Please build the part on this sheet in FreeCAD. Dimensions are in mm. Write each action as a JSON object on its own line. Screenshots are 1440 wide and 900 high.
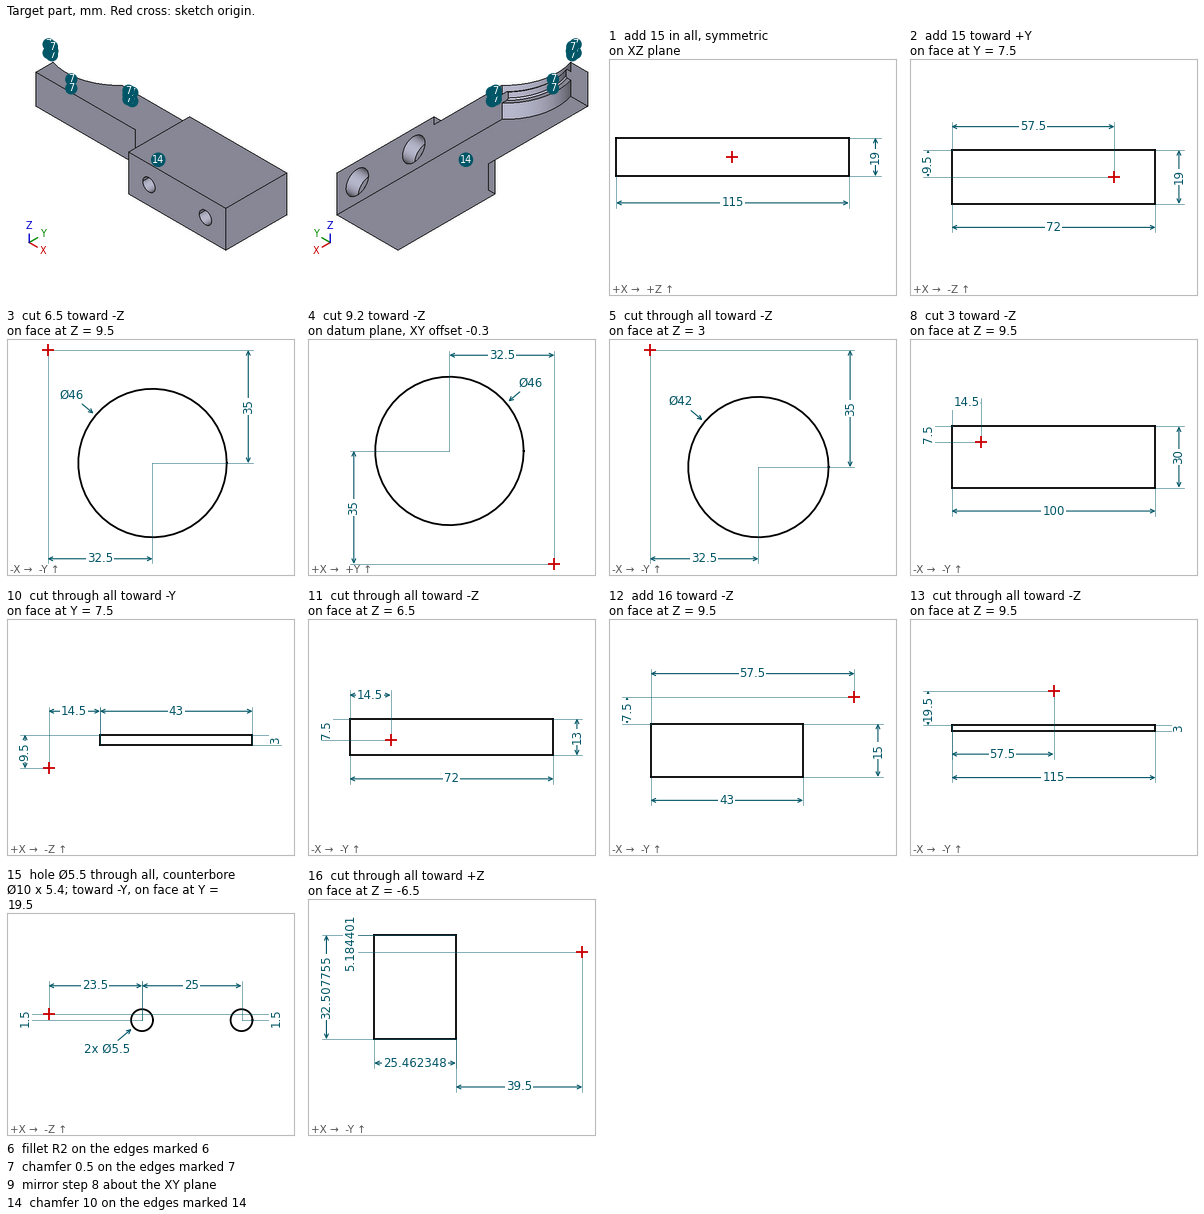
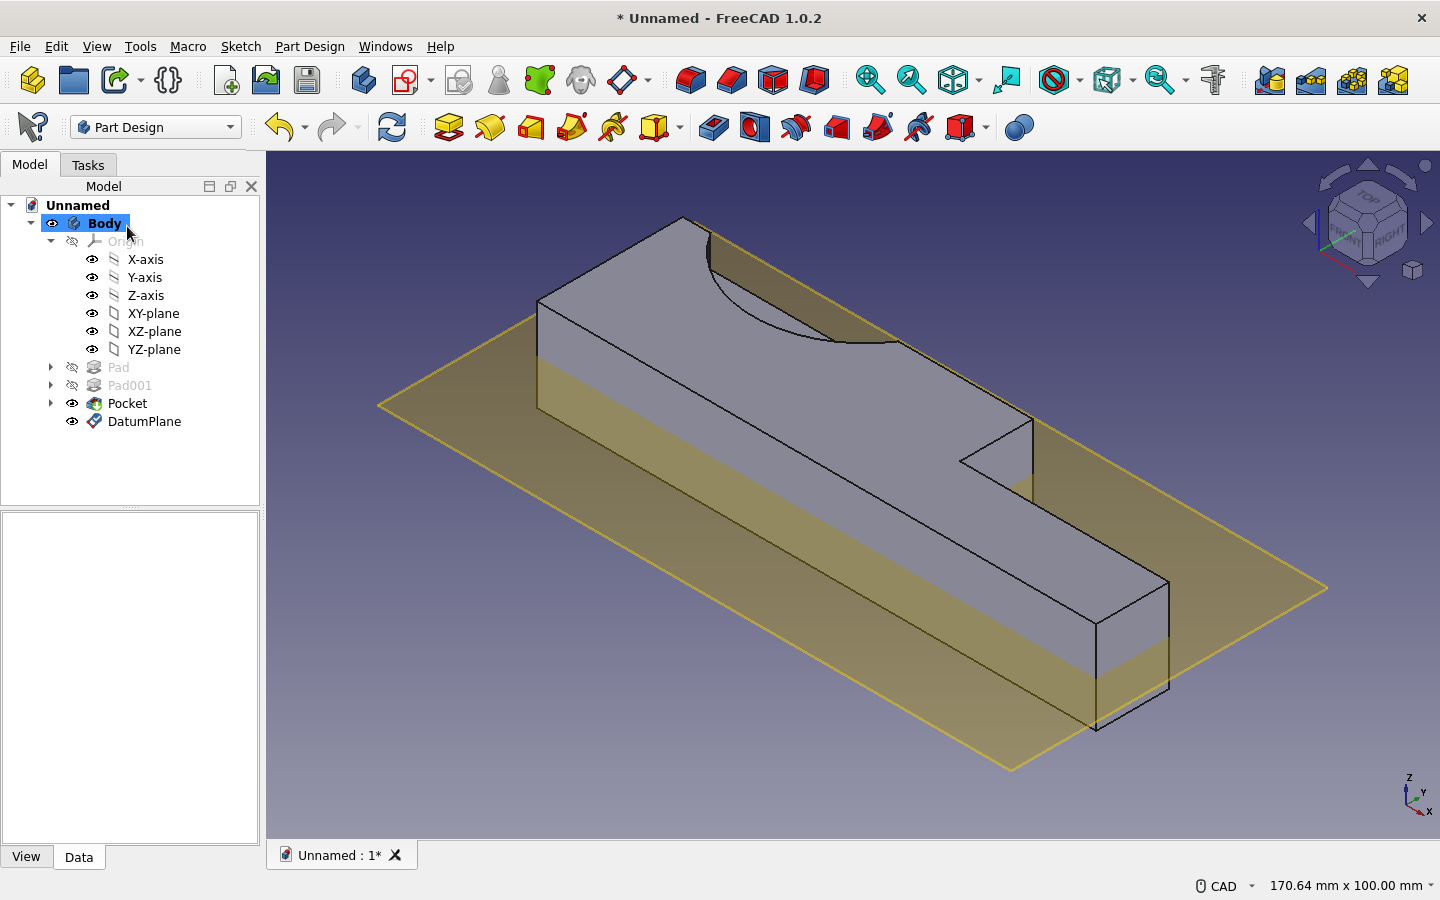
{"action": "left_click", "coordinate": [117, 421]}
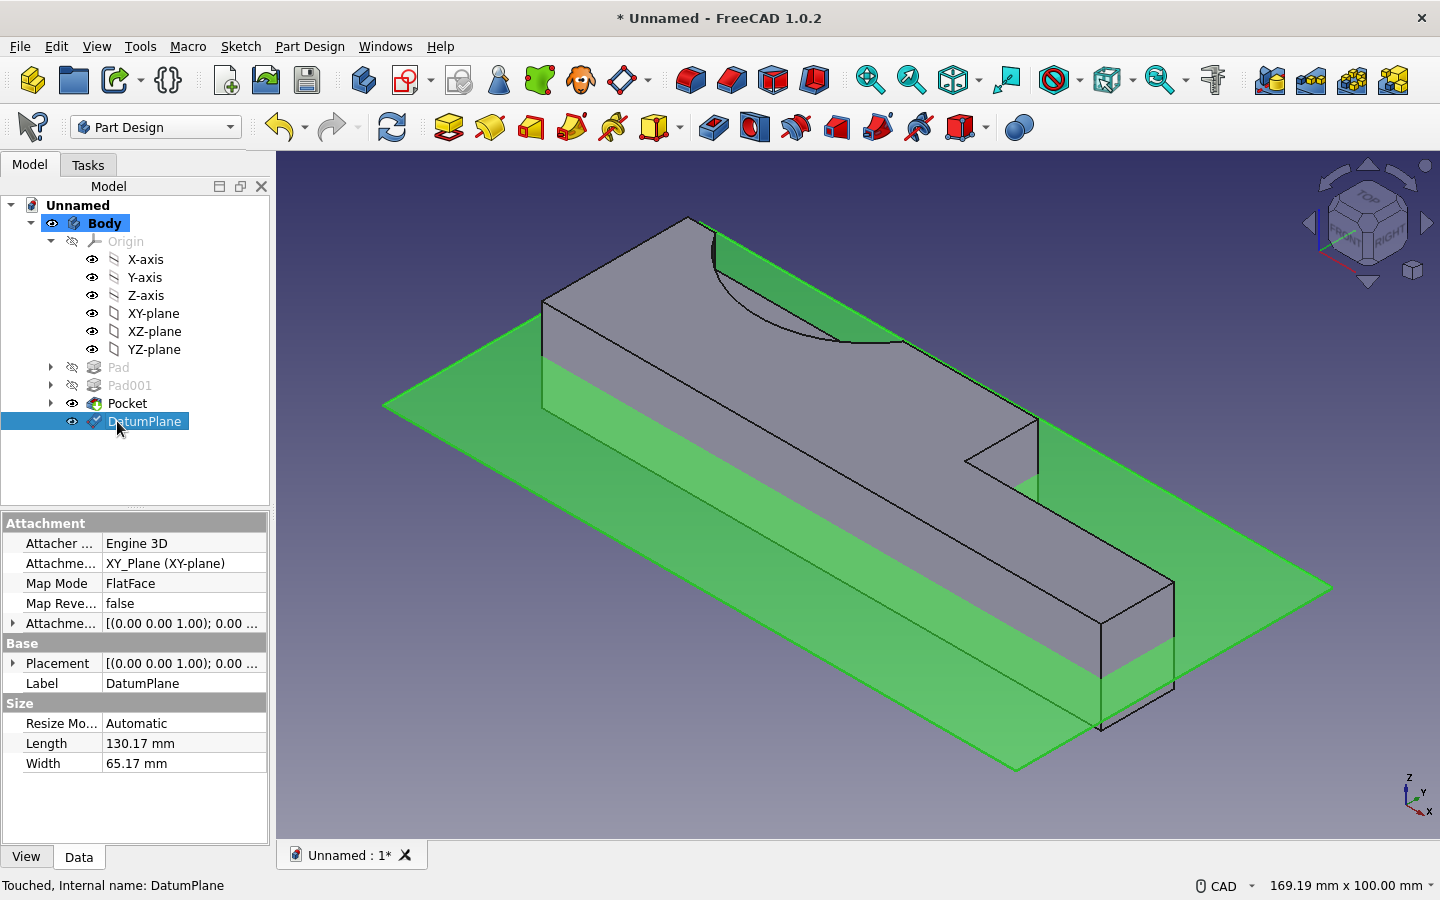
{"action": "left_click", "coordinate": [404, 80]}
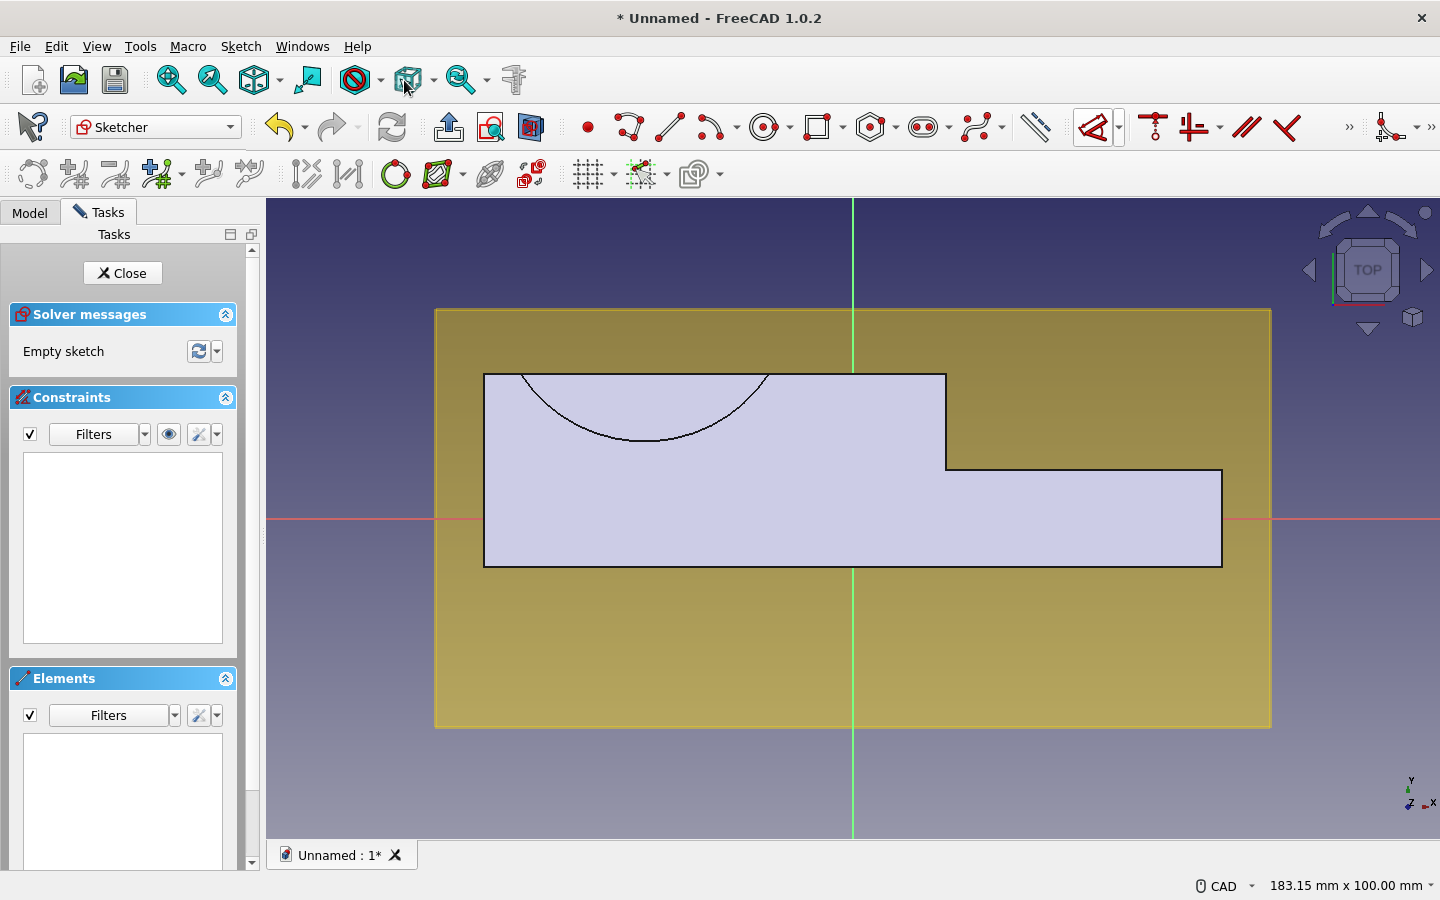
{"action": "left_click", "coordinate": [531, 128]}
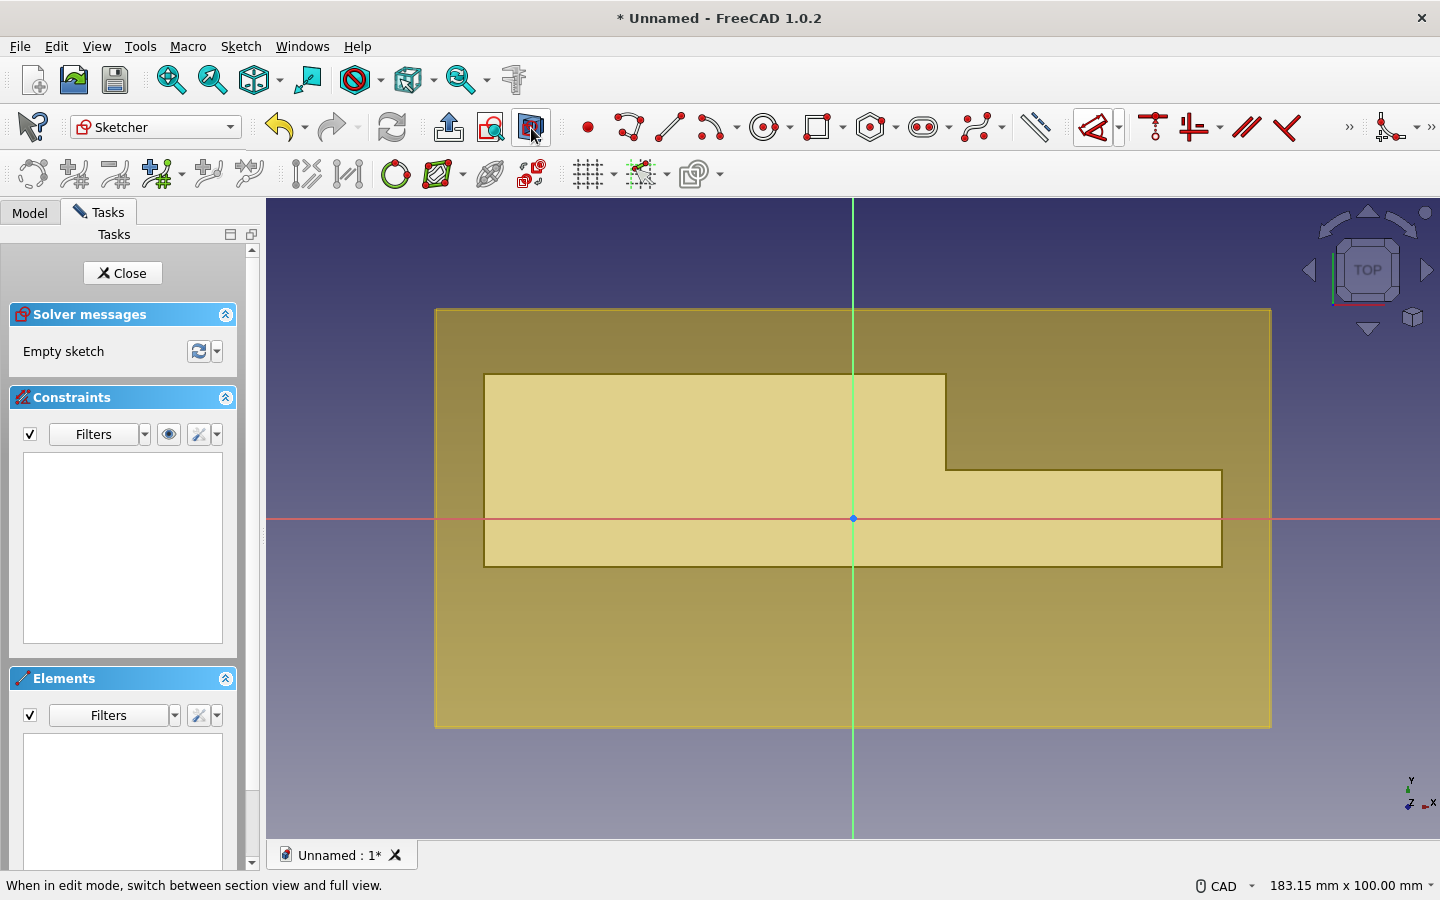
{"action": "scroll", "coordinate": [1275, 811], "scroll_direction": "down", "scroll_amount": 1}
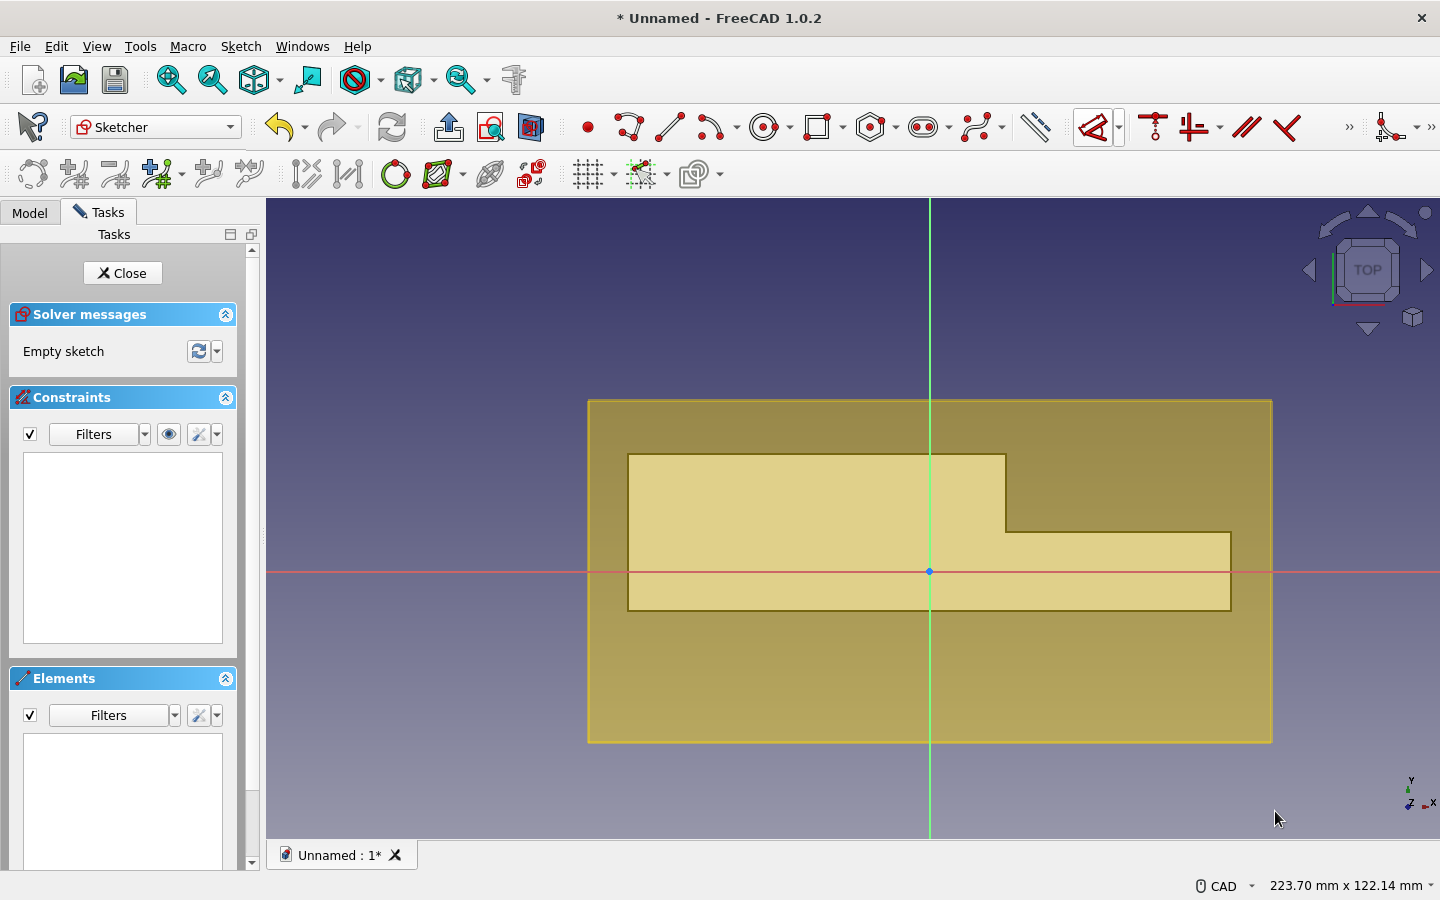
{"action": "scroll", "coordinate": [783, 226], "scroll_direction": "up", "scroll_amount": 2}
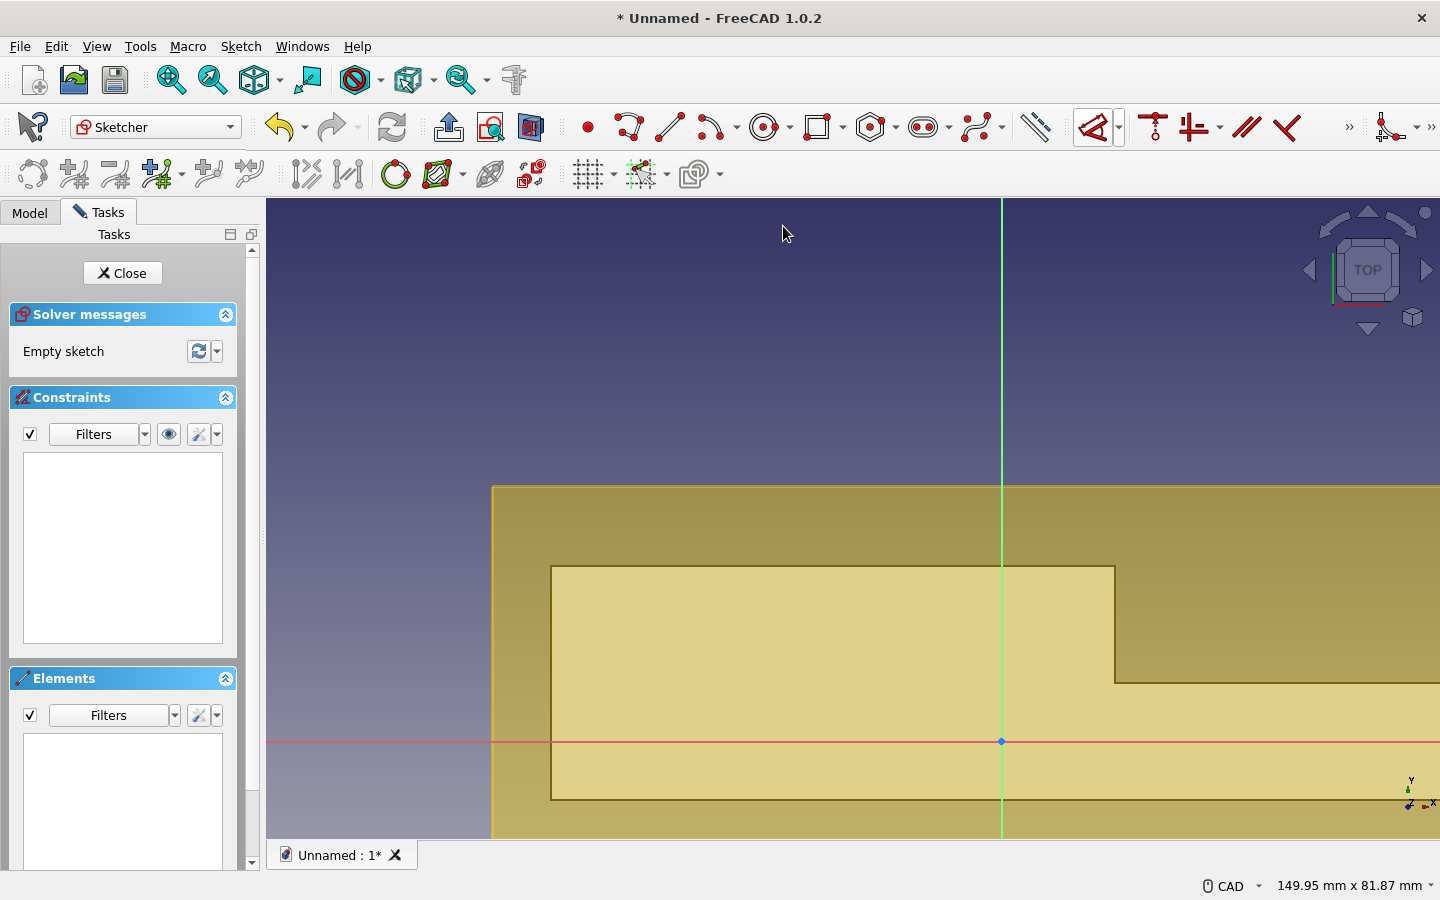
{"action": "left_click", "coordinate": [764, 128]}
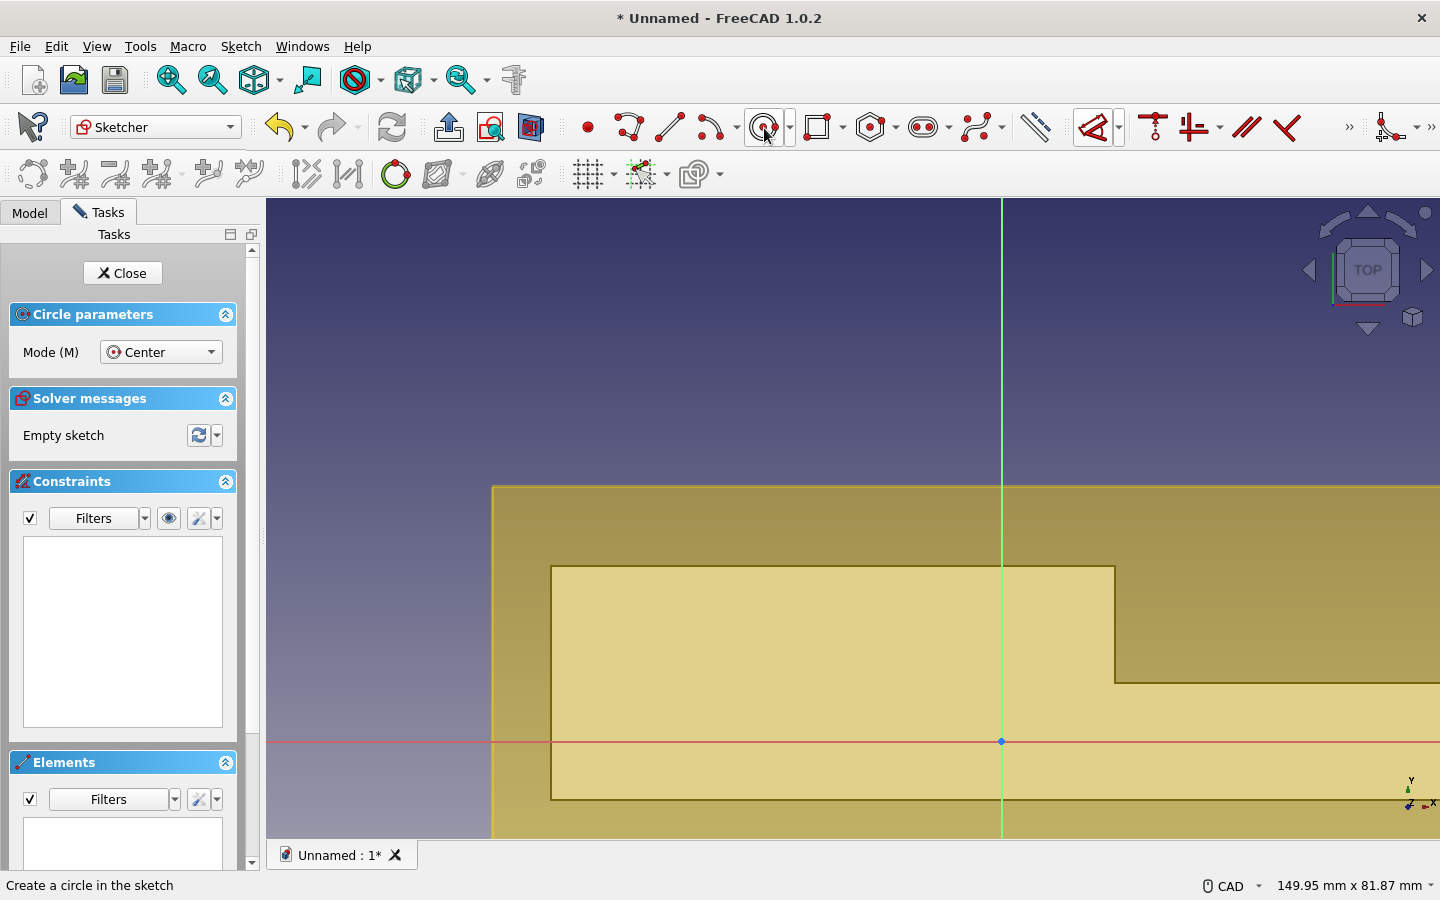
{"action": "left_click", "coordinate": [747, 468]}
{"action": "mouse_move", "coordinate": [874, 340]}